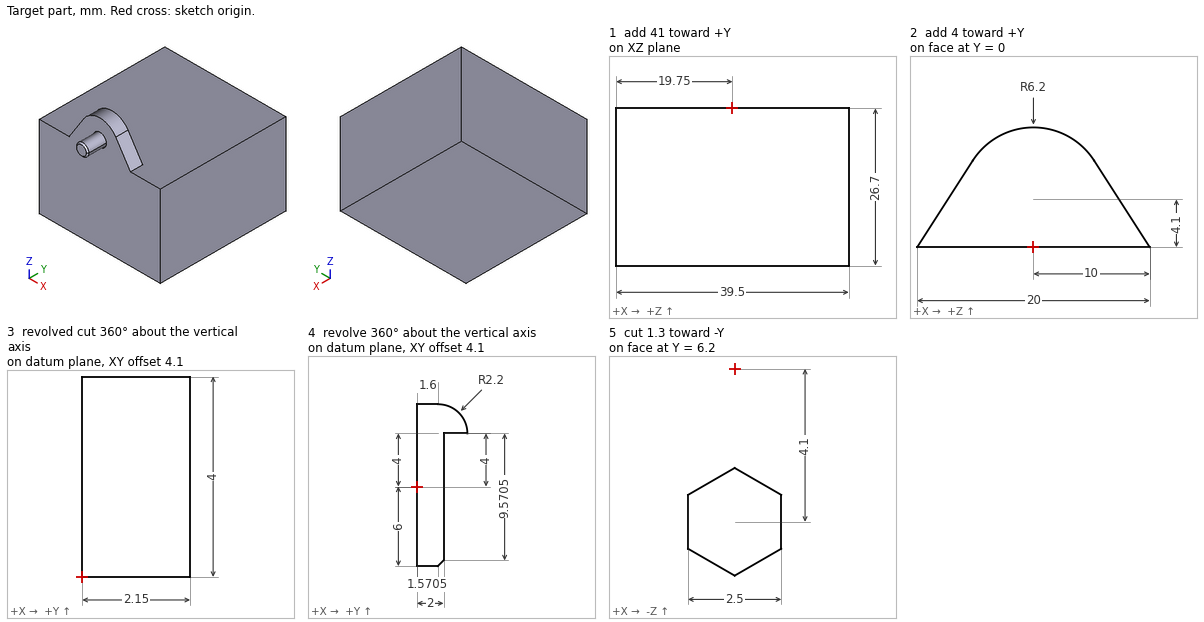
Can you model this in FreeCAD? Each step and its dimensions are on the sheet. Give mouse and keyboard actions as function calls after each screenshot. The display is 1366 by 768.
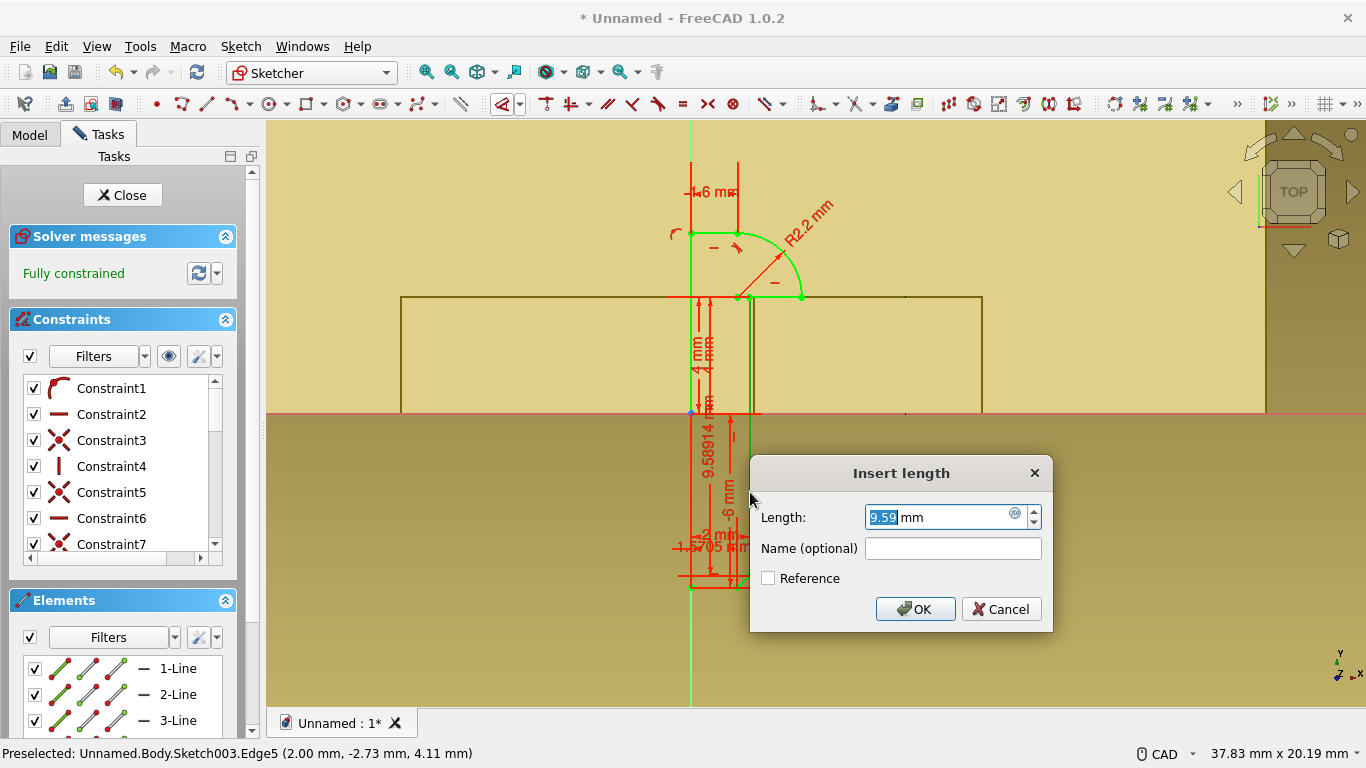
text(9.5705)
key(Return)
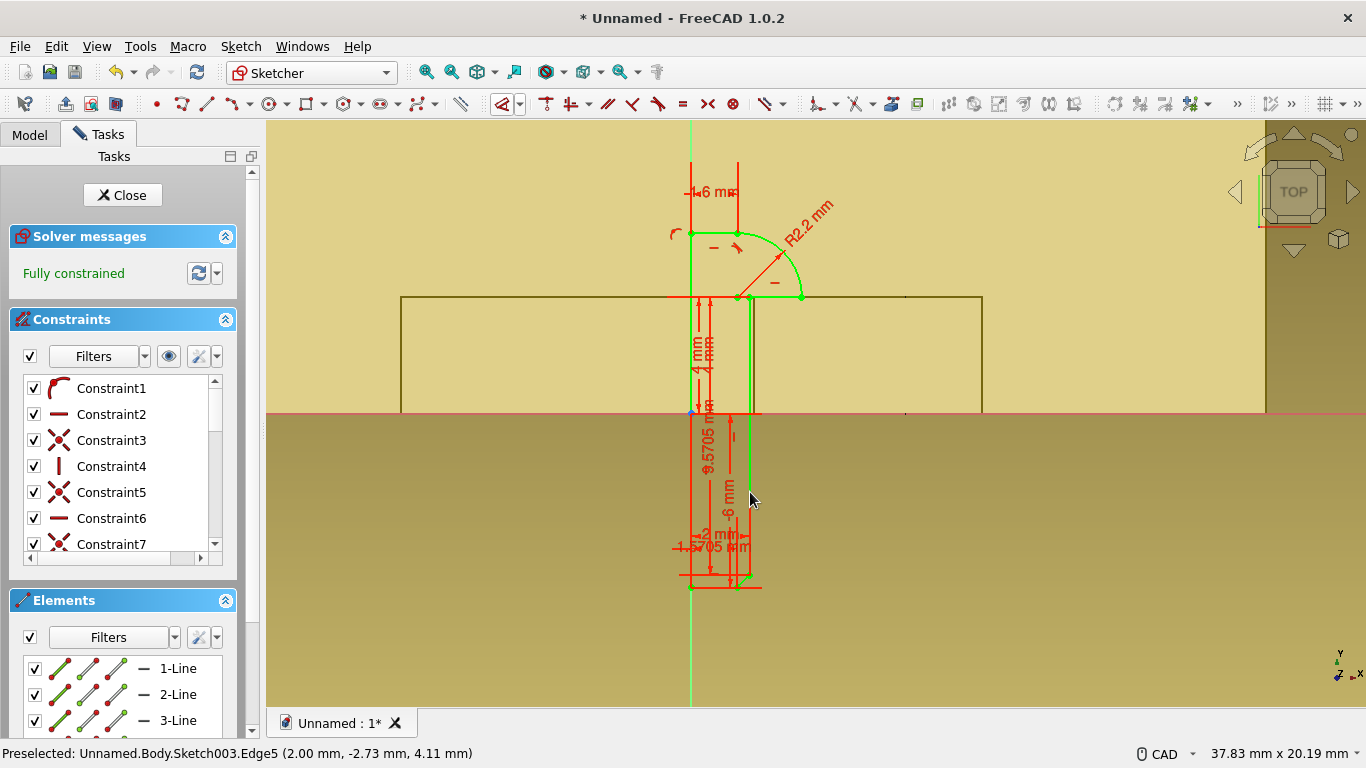
click(123, 195)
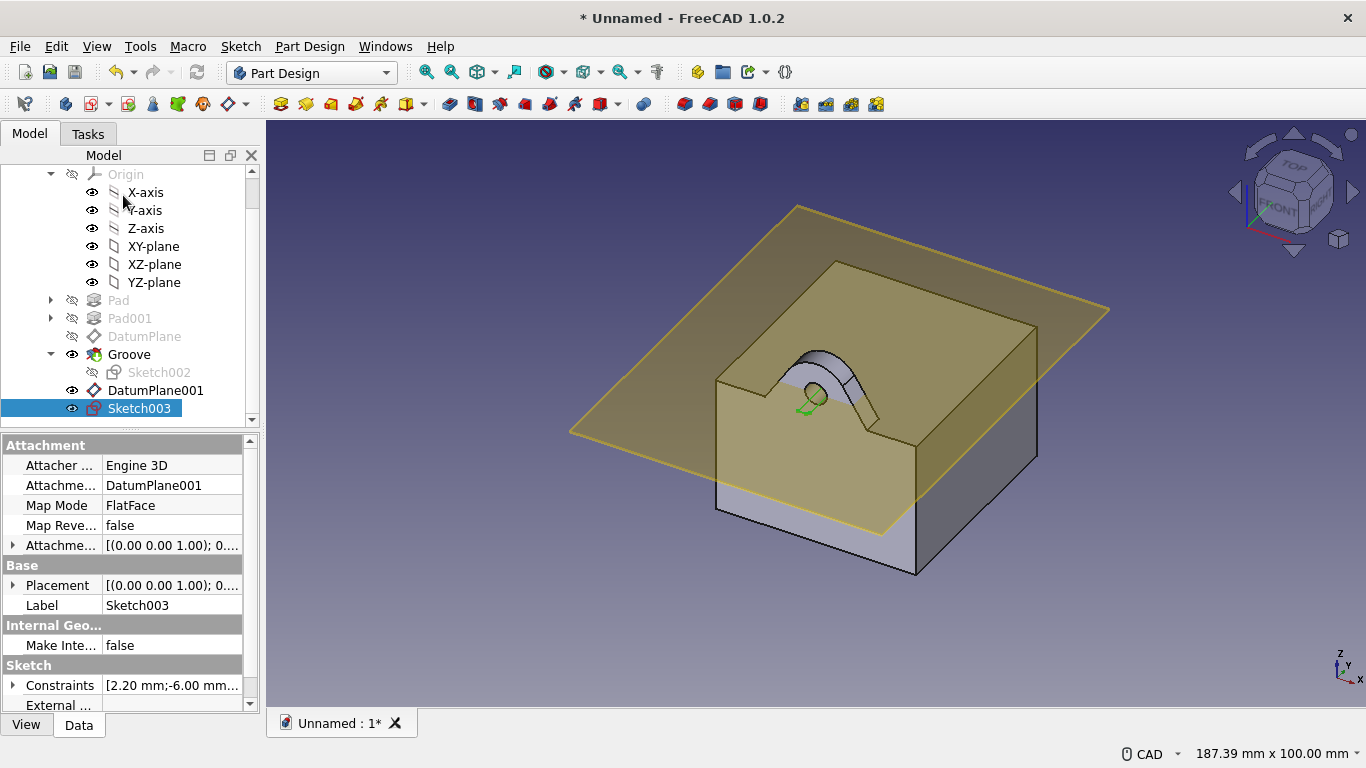
click(306, 104)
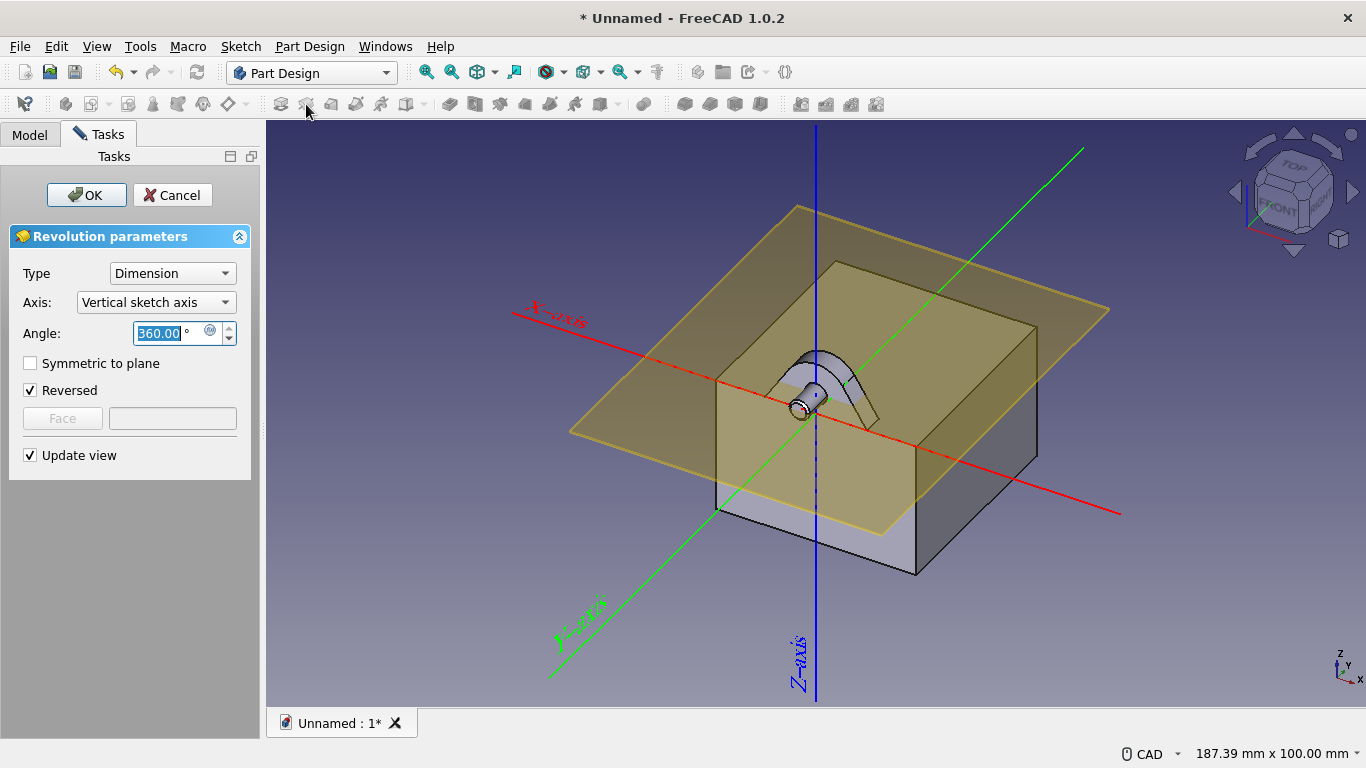
click(87, 195)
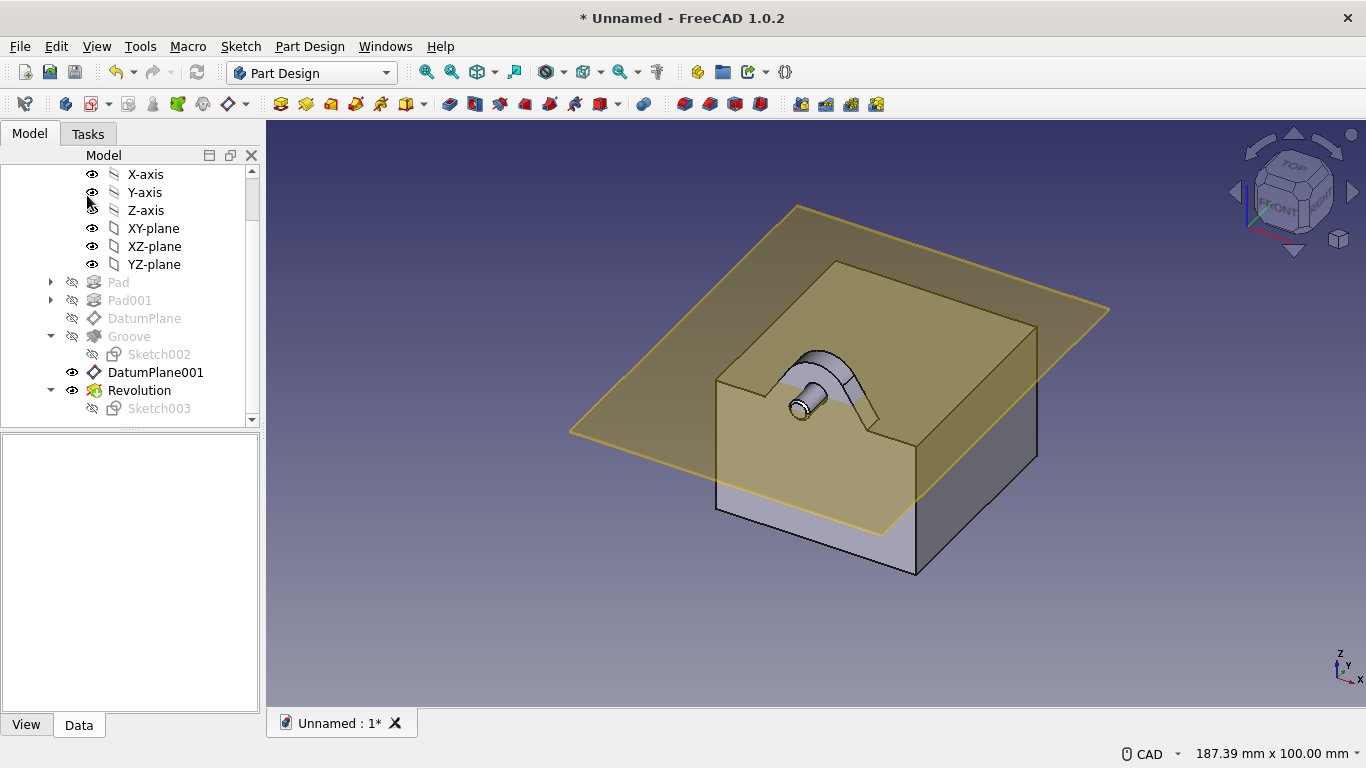
click(117, 372)
key(space)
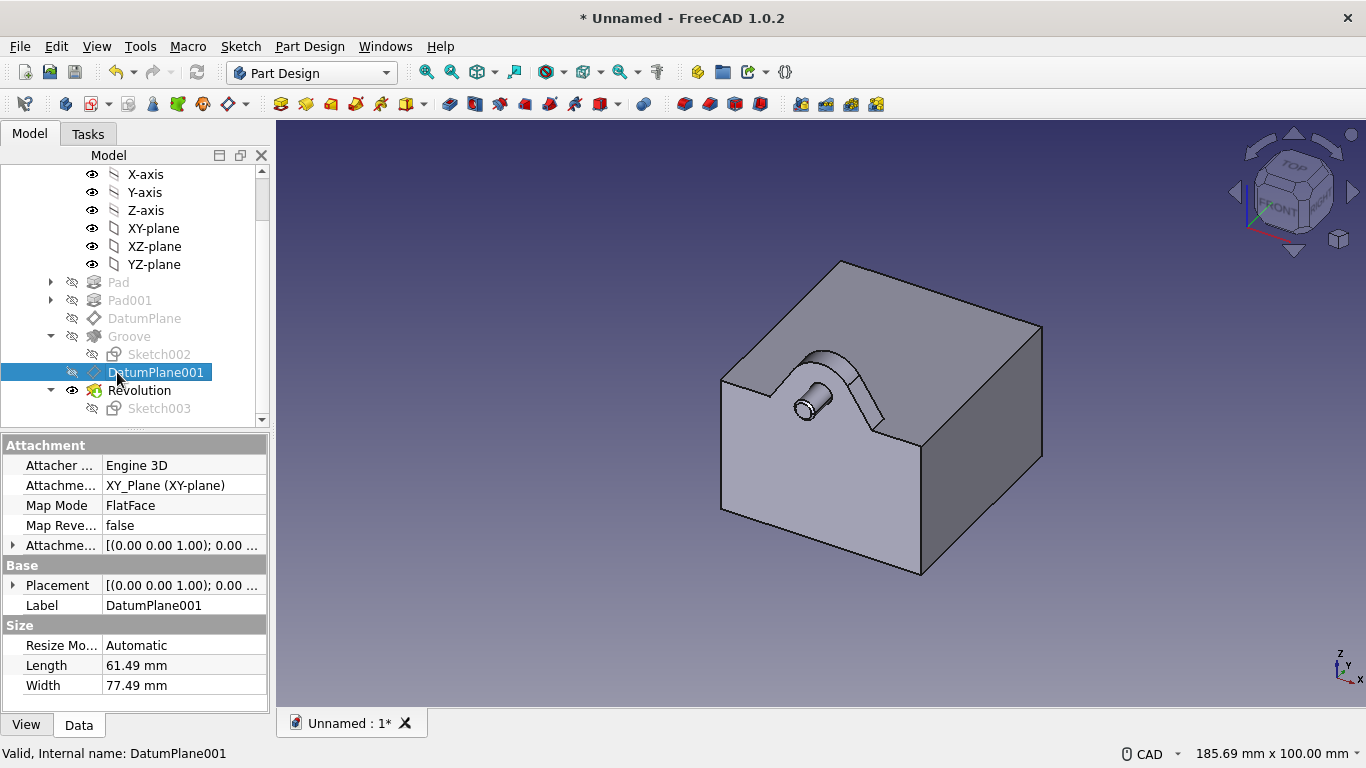
key(4)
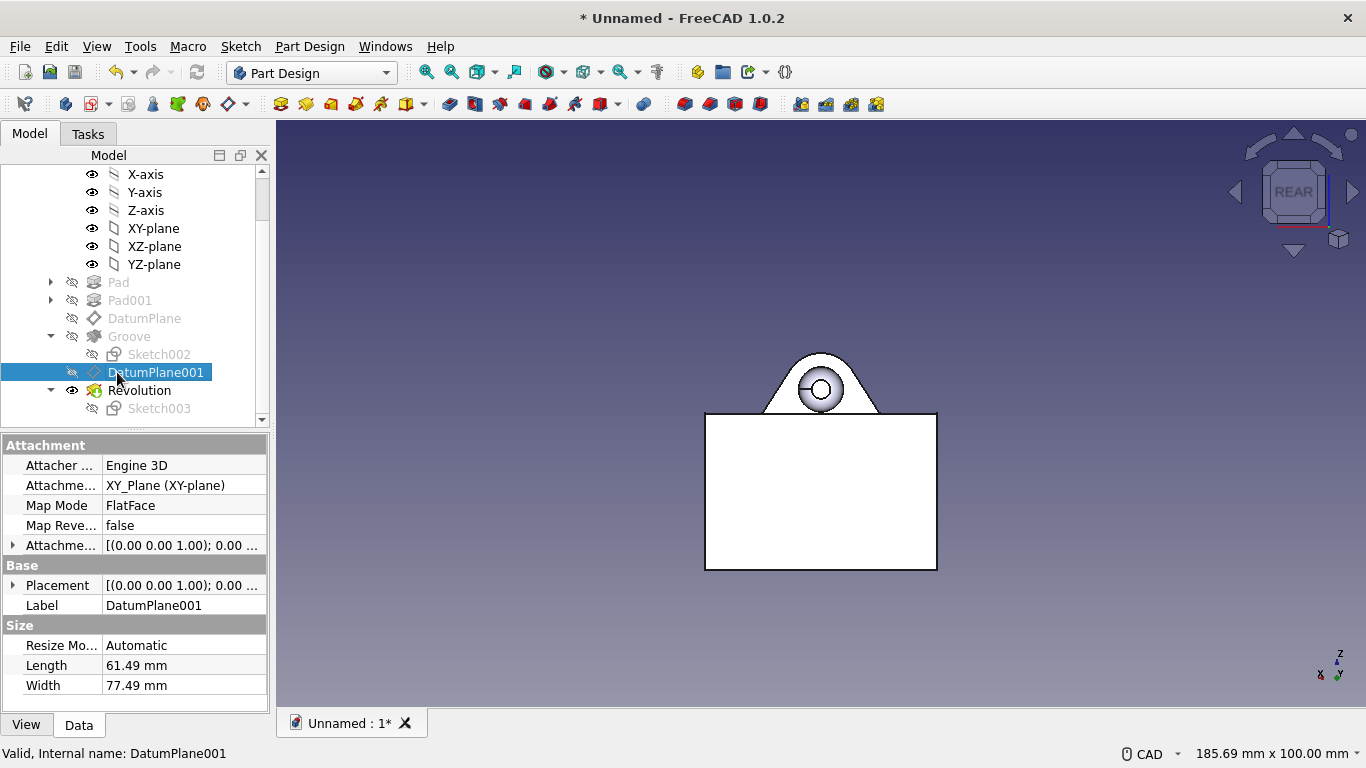
click(427, 72)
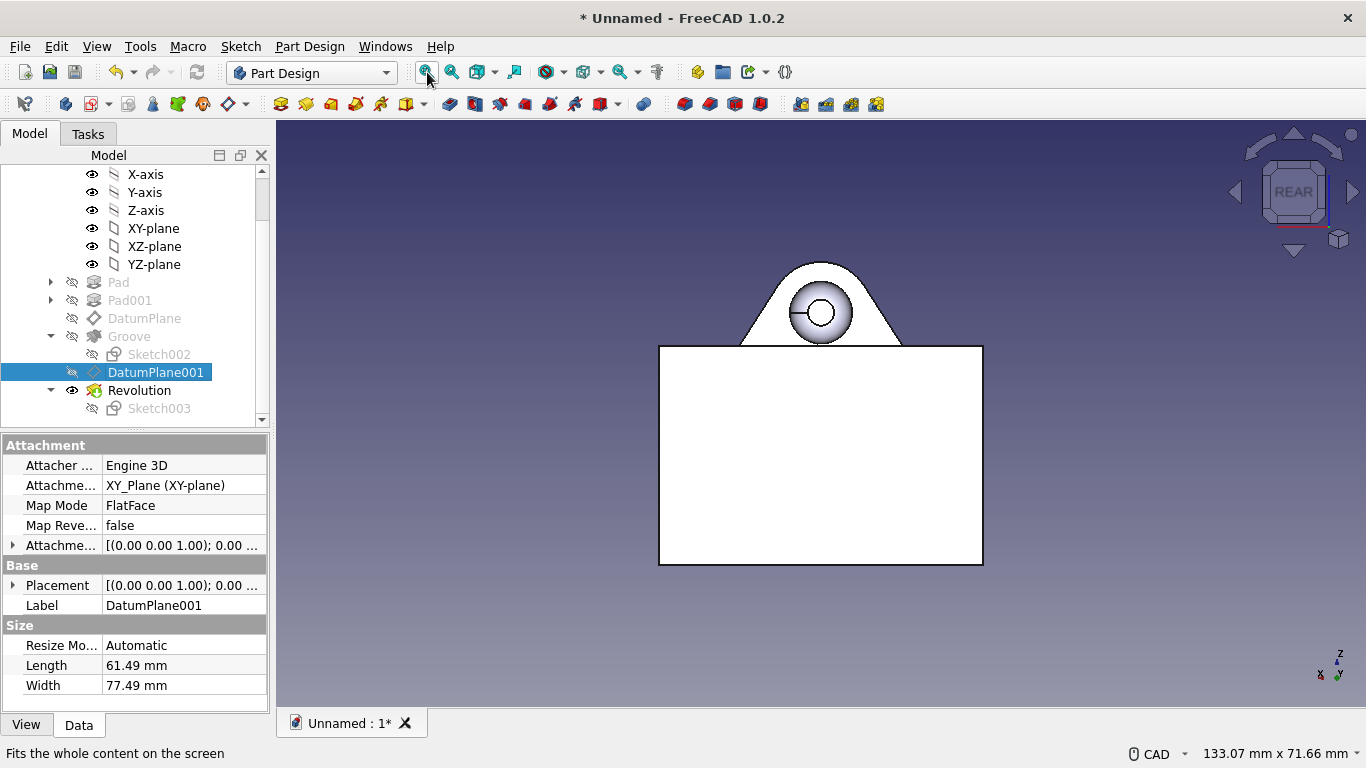
click(821, 312)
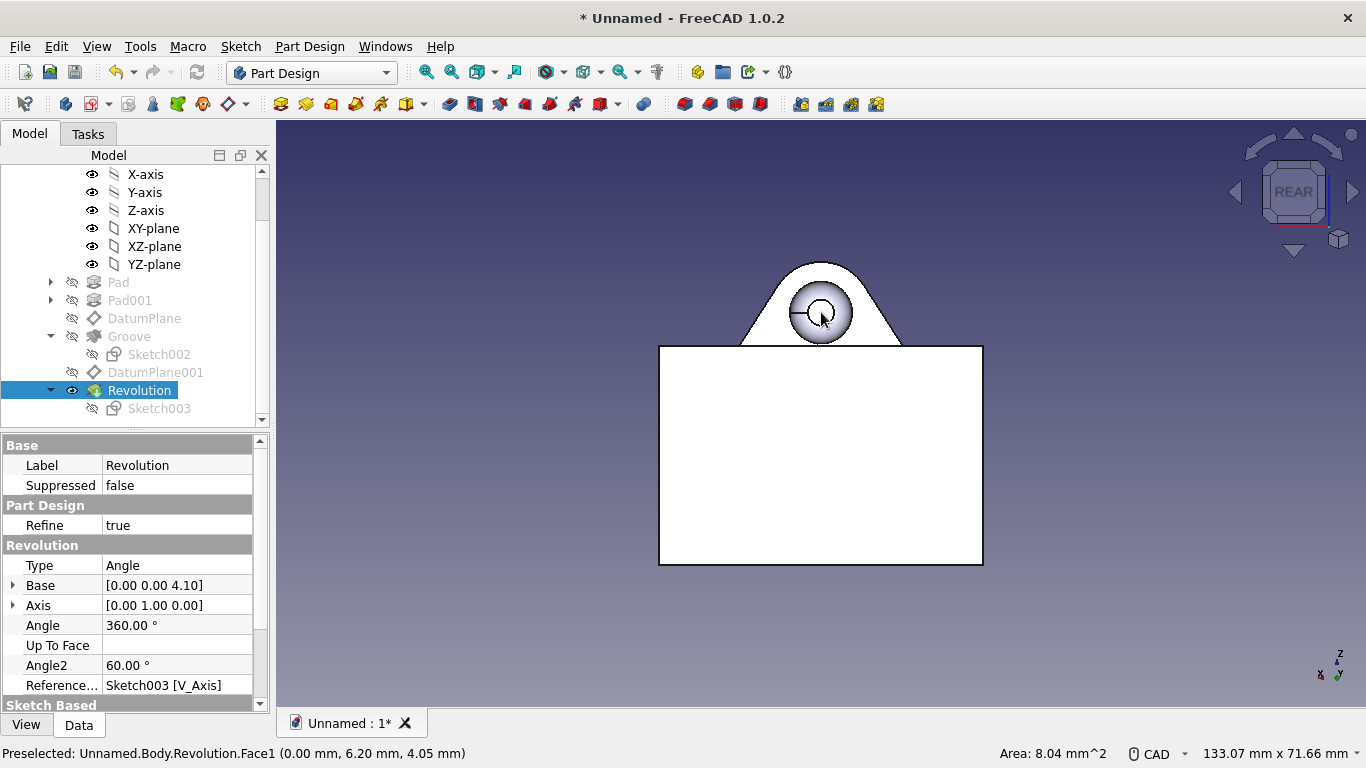
click(90, 104)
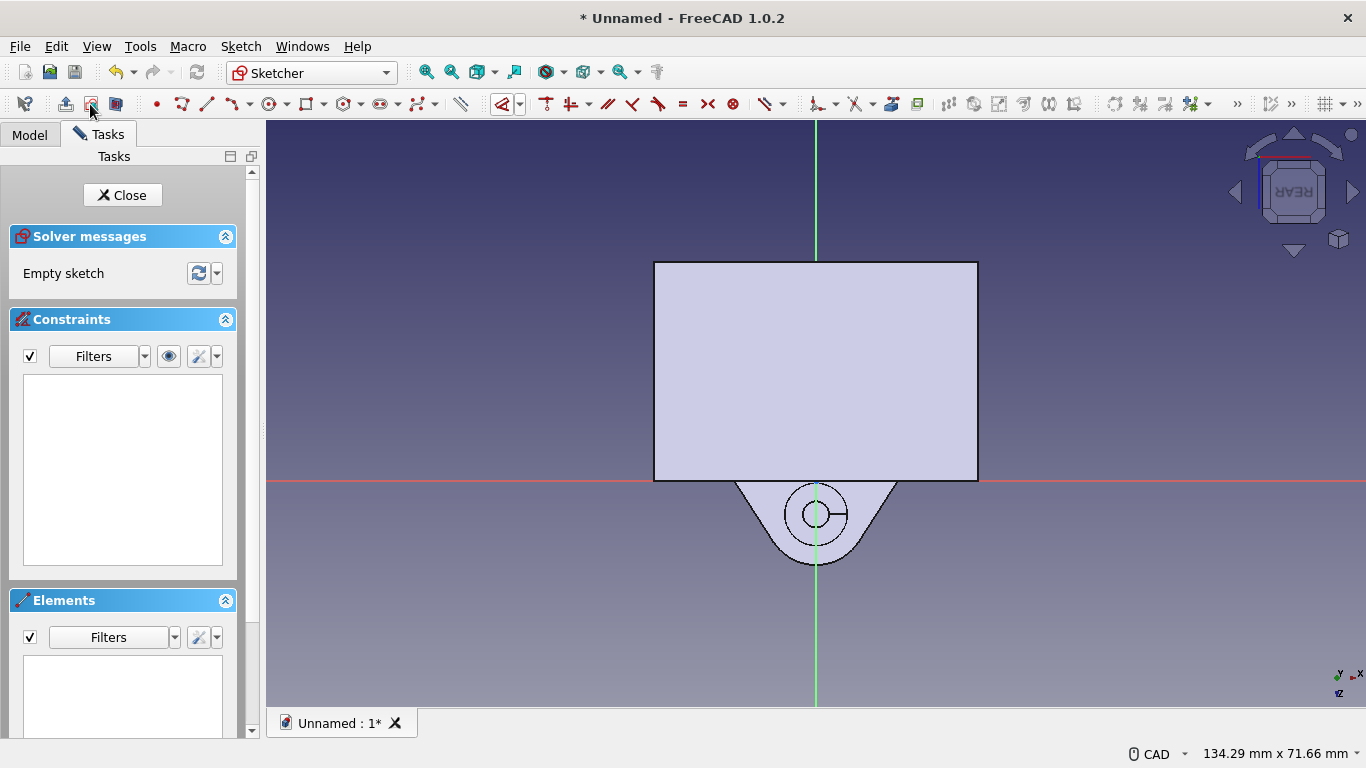
click(116, 104)